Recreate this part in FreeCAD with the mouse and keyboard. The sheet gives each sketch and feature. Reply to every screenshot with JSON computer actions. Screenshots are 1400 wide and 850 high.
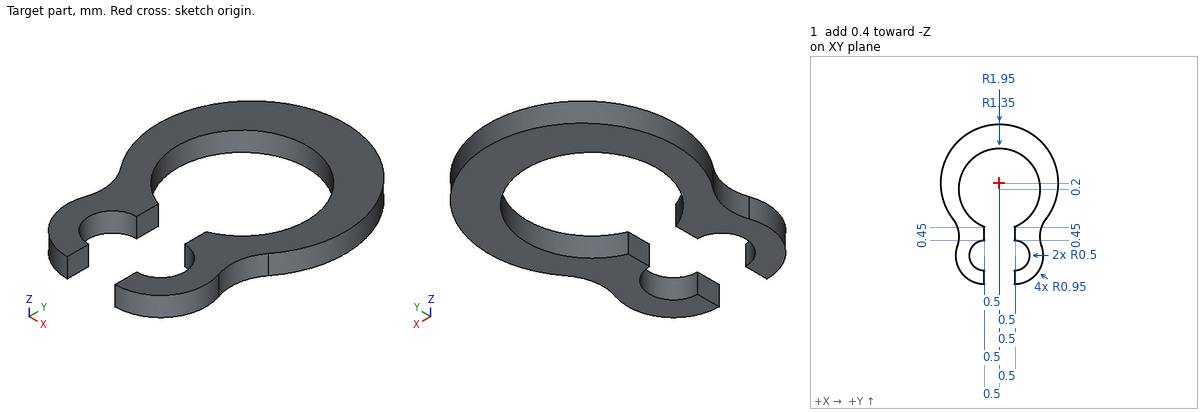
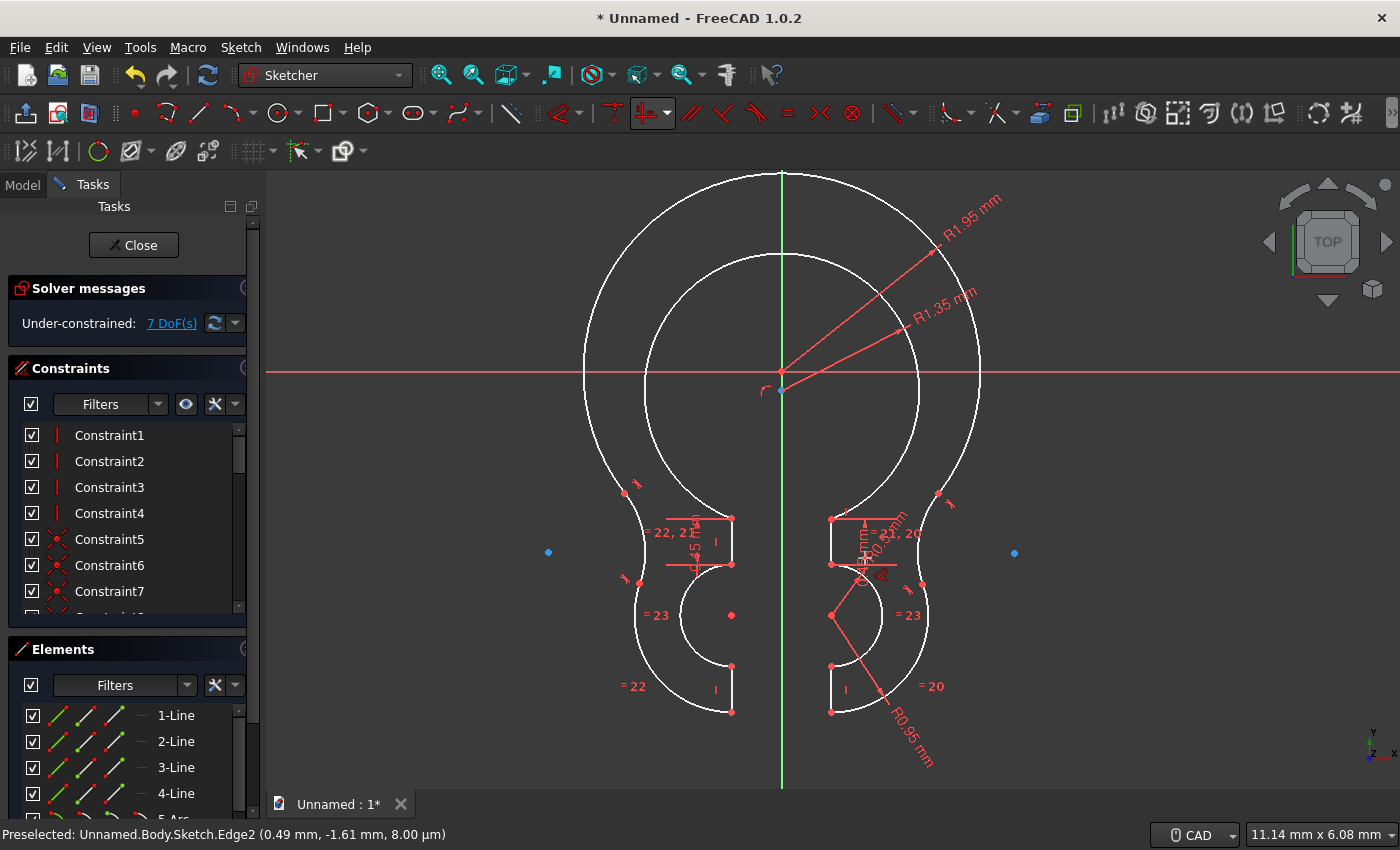
{"action": "left_click", "coordinate": [732, 565]}
{"action": "left_click", "coordinate": [757, 599]}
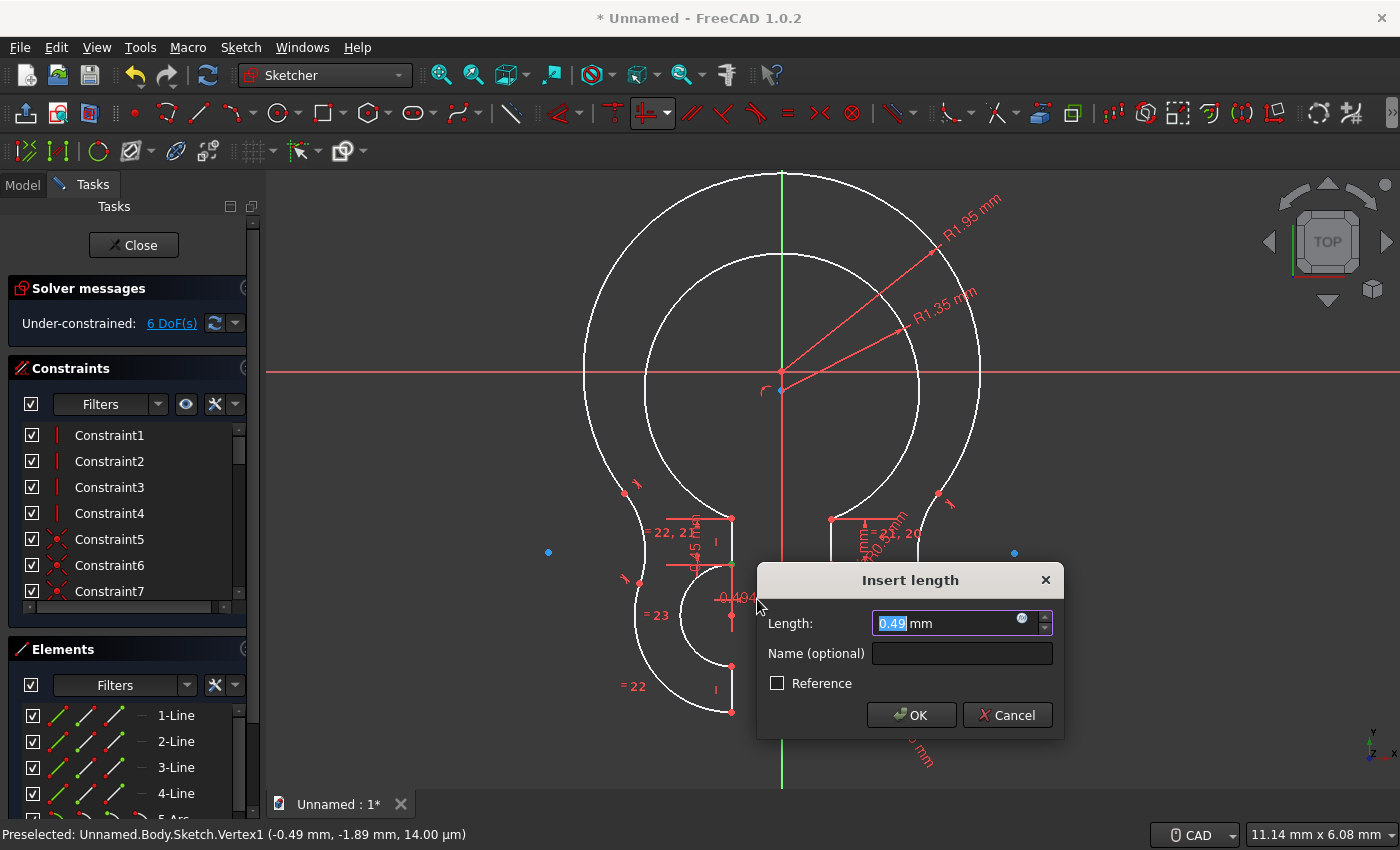
{"action": "type", "text": "0.5"}
{"action": "key", "text": "Return"}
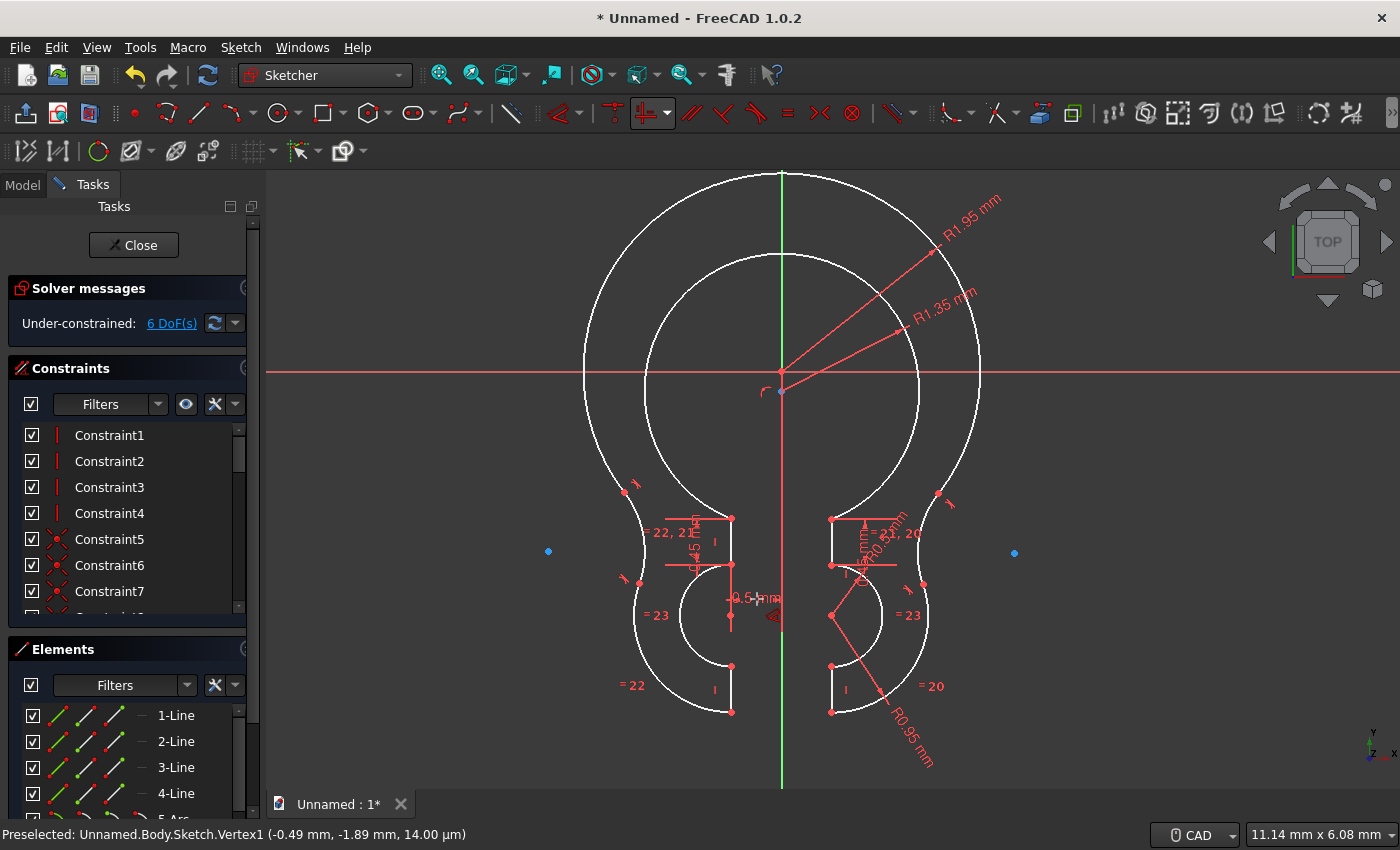
{"action": "left_click", "coordinate": [832, 519]}
{"action": "left_click", "coordinate": [795, 553]}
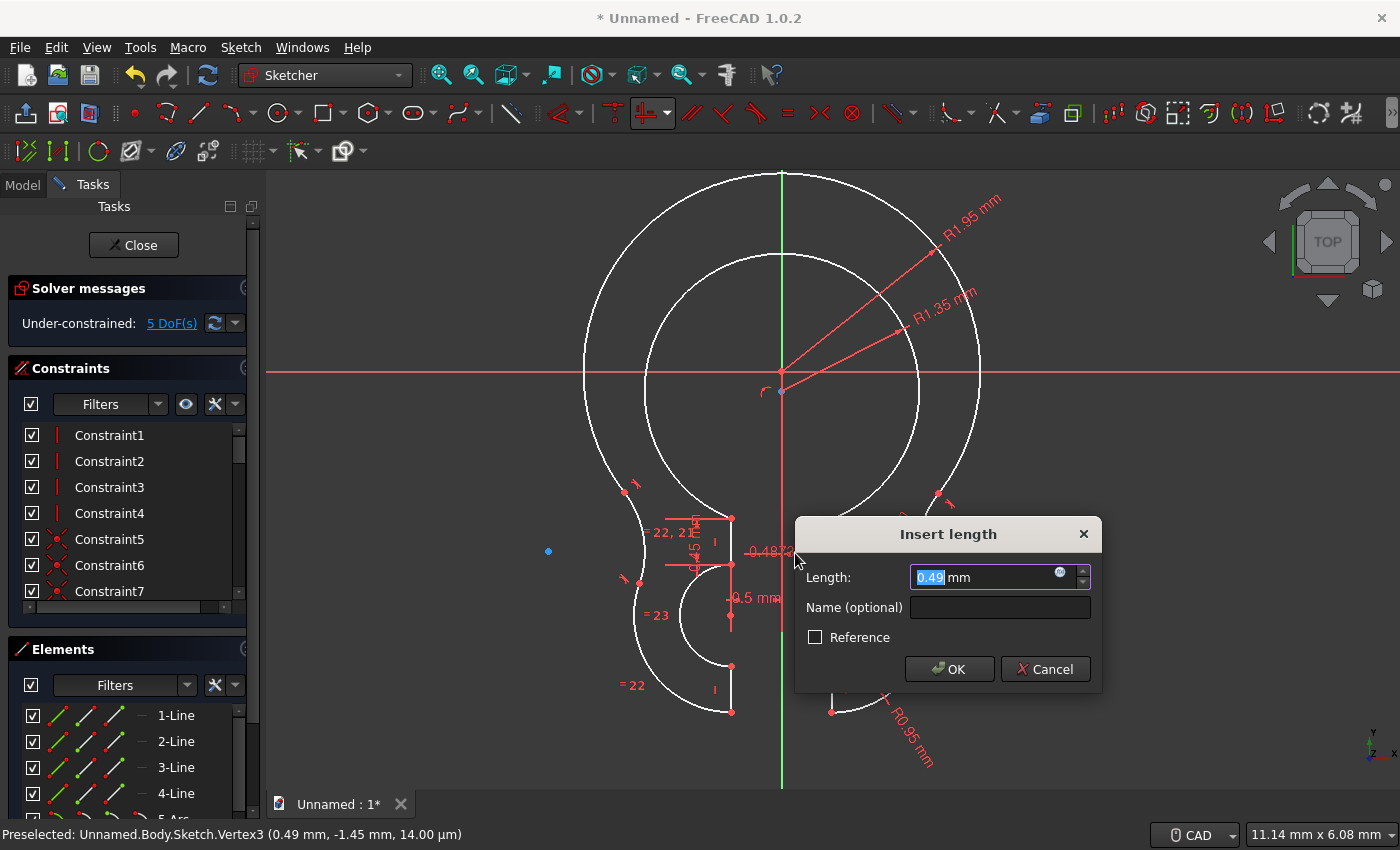
{"action": "type", "text": "0.5"}
{"action": "key", "text": "Return"}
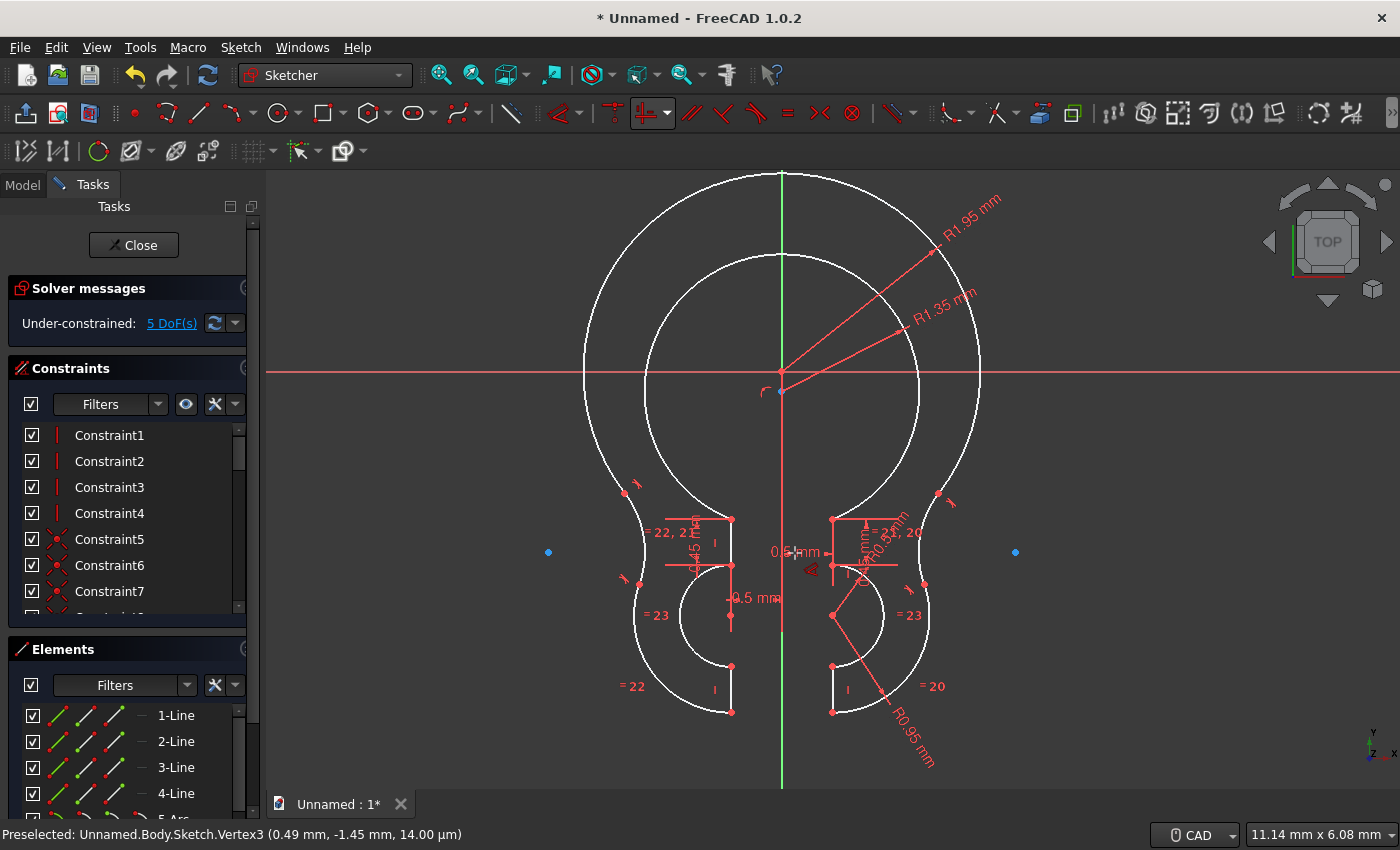
{"action": "left_click", "coordinate": [833, 667]}
{"action": "left_click", "coordinate": [807, 701]}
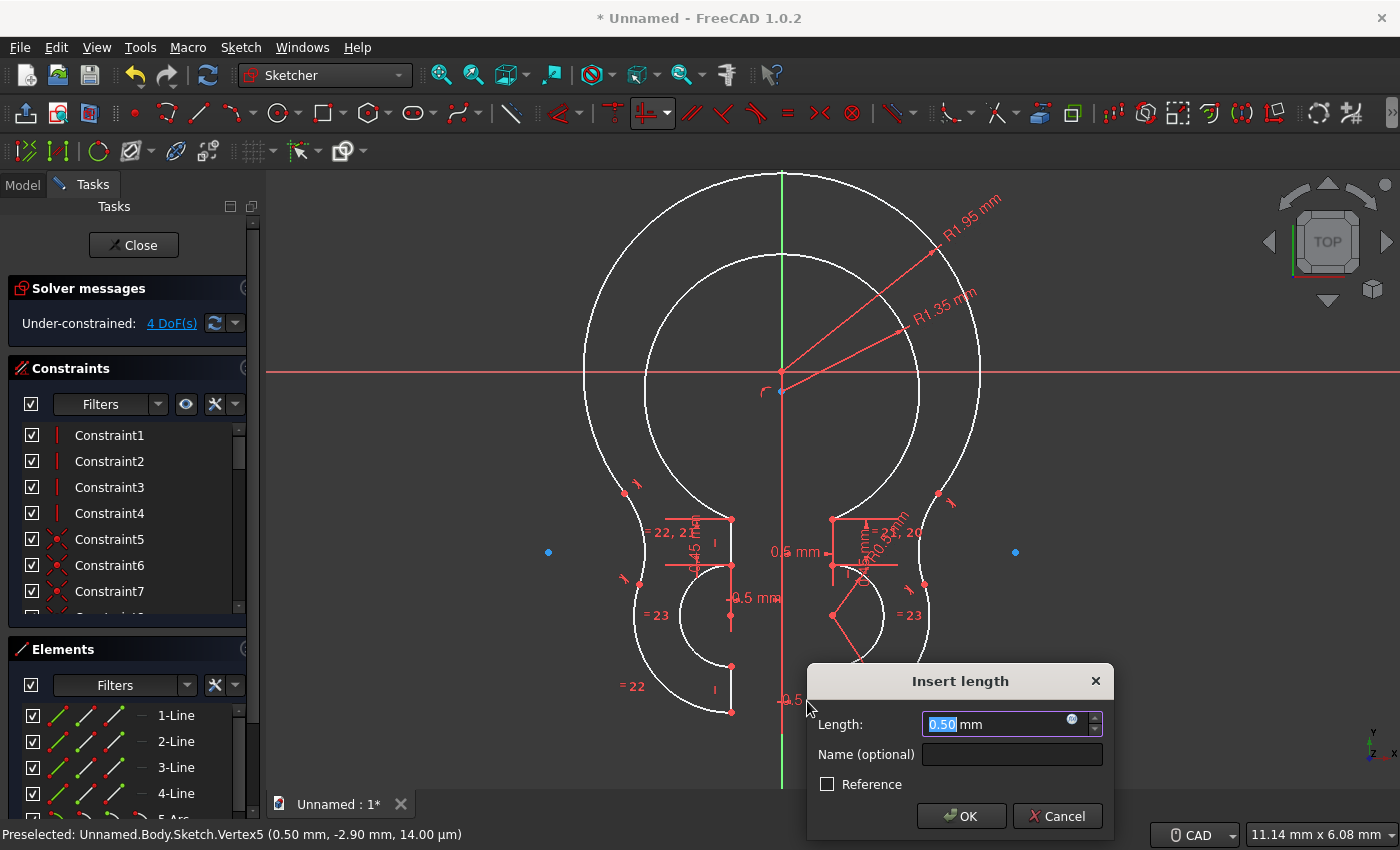
{"action": "type", "text": "0.5"}
{"action": "key", "text": "Return"}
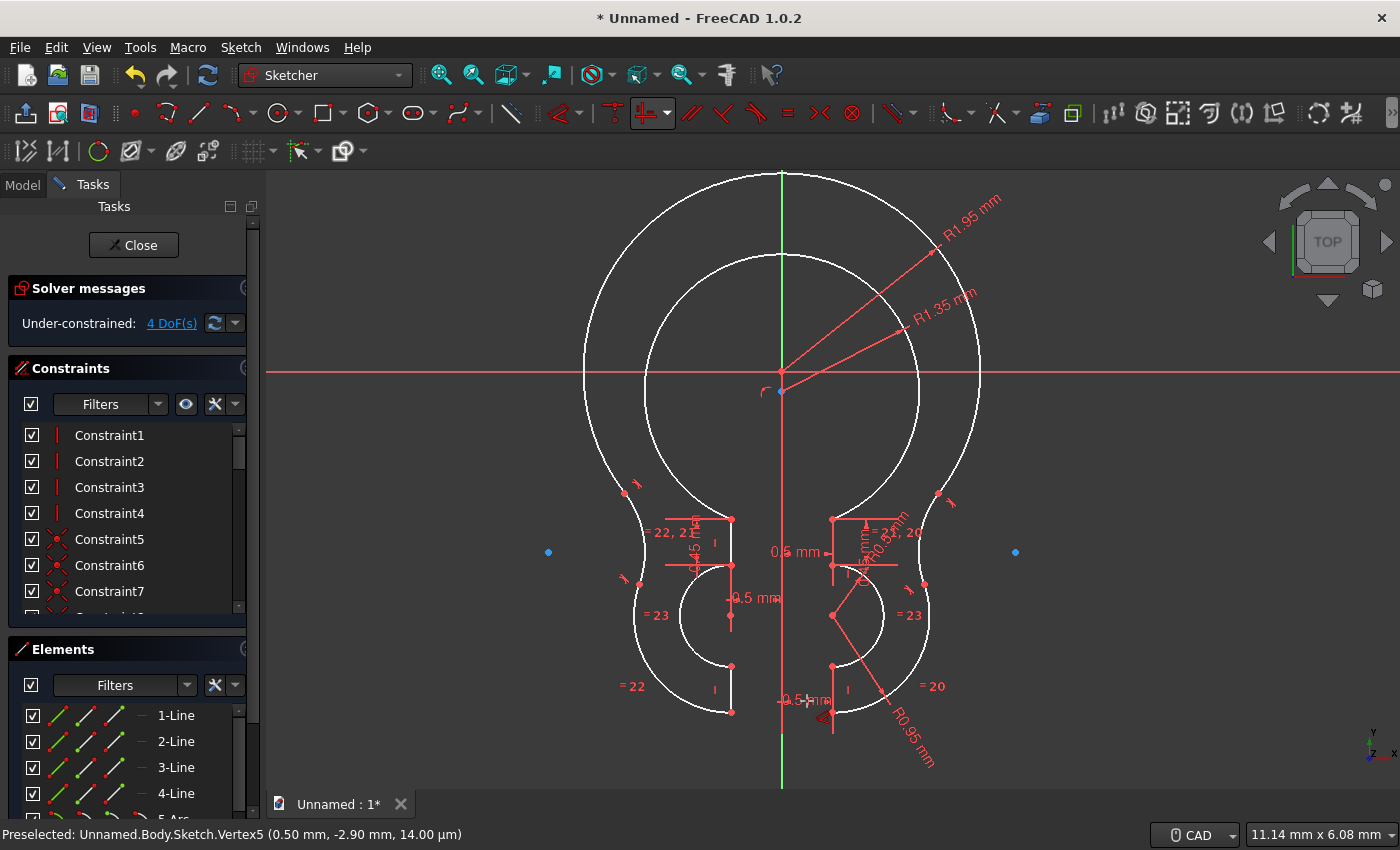
{"action": "left_click", "coordinate": [731, 713]}
{"action": "left_click", "coordinate": [756, 747]}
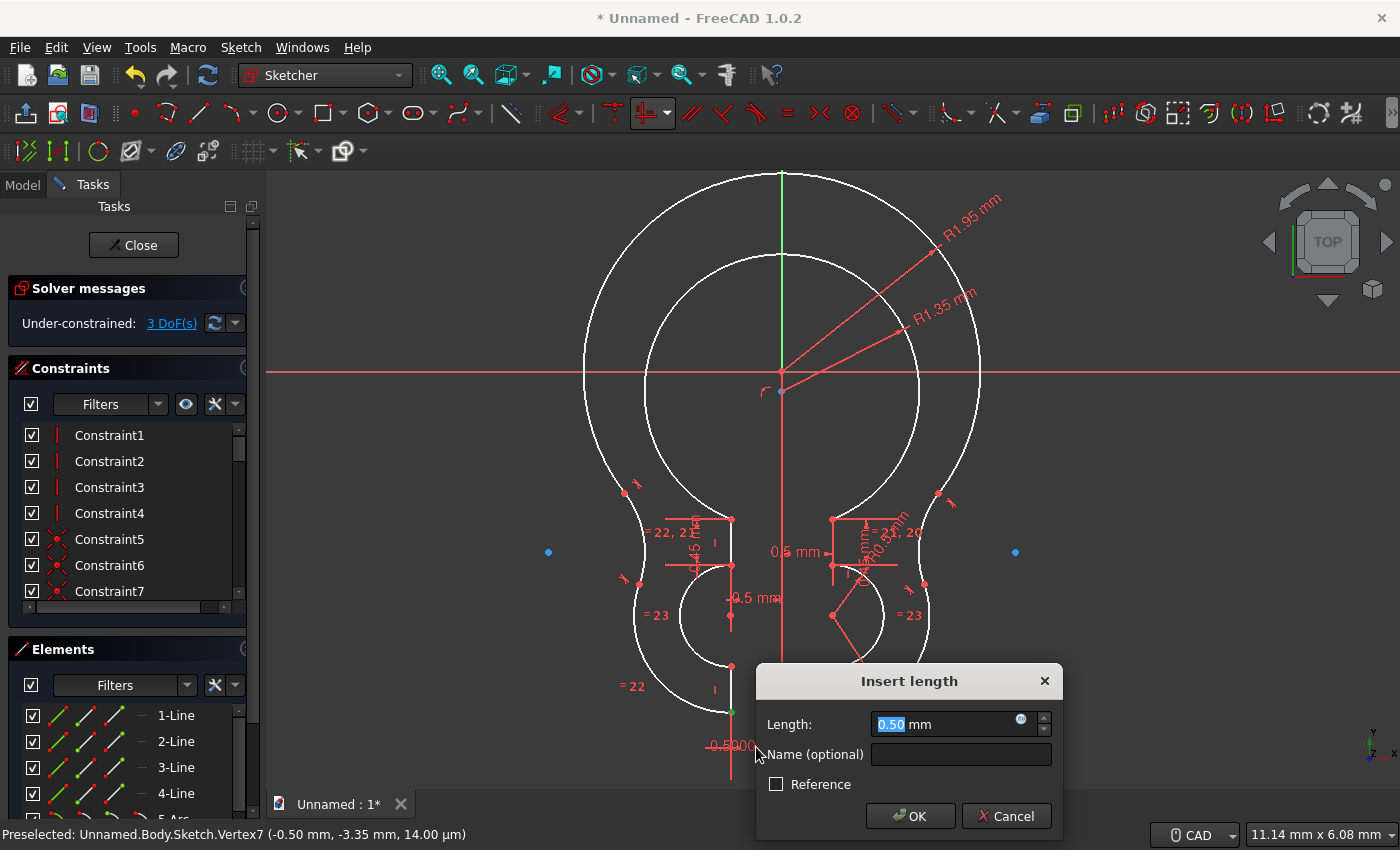
{"action": "type", "text": "0.5"}
{"action": "key", "text": "Return"}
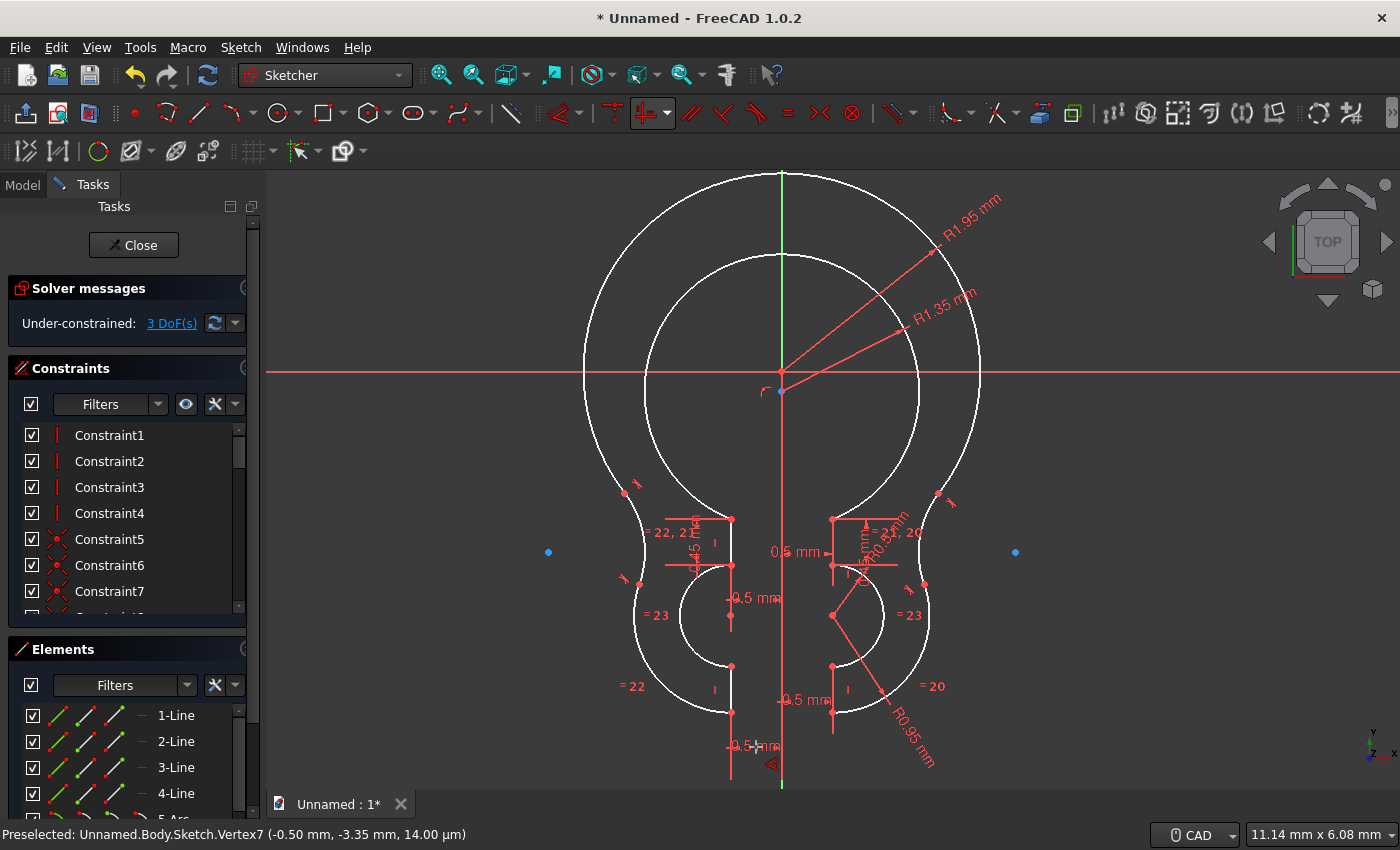
{"action": "scroll", "coordinate": [782, 392], "scroll_direction": "up", "scroll_amount": 4}